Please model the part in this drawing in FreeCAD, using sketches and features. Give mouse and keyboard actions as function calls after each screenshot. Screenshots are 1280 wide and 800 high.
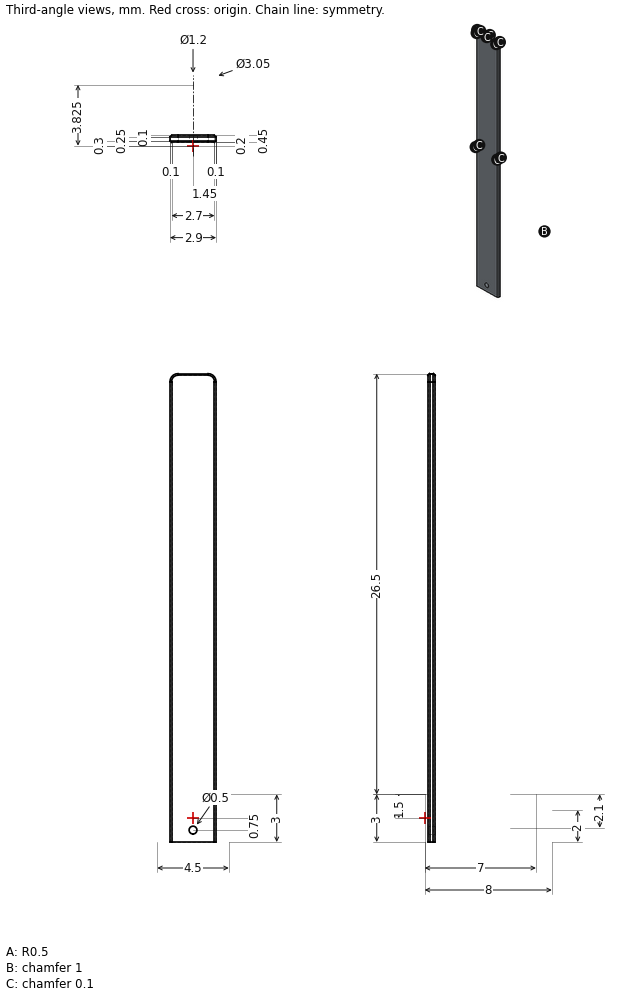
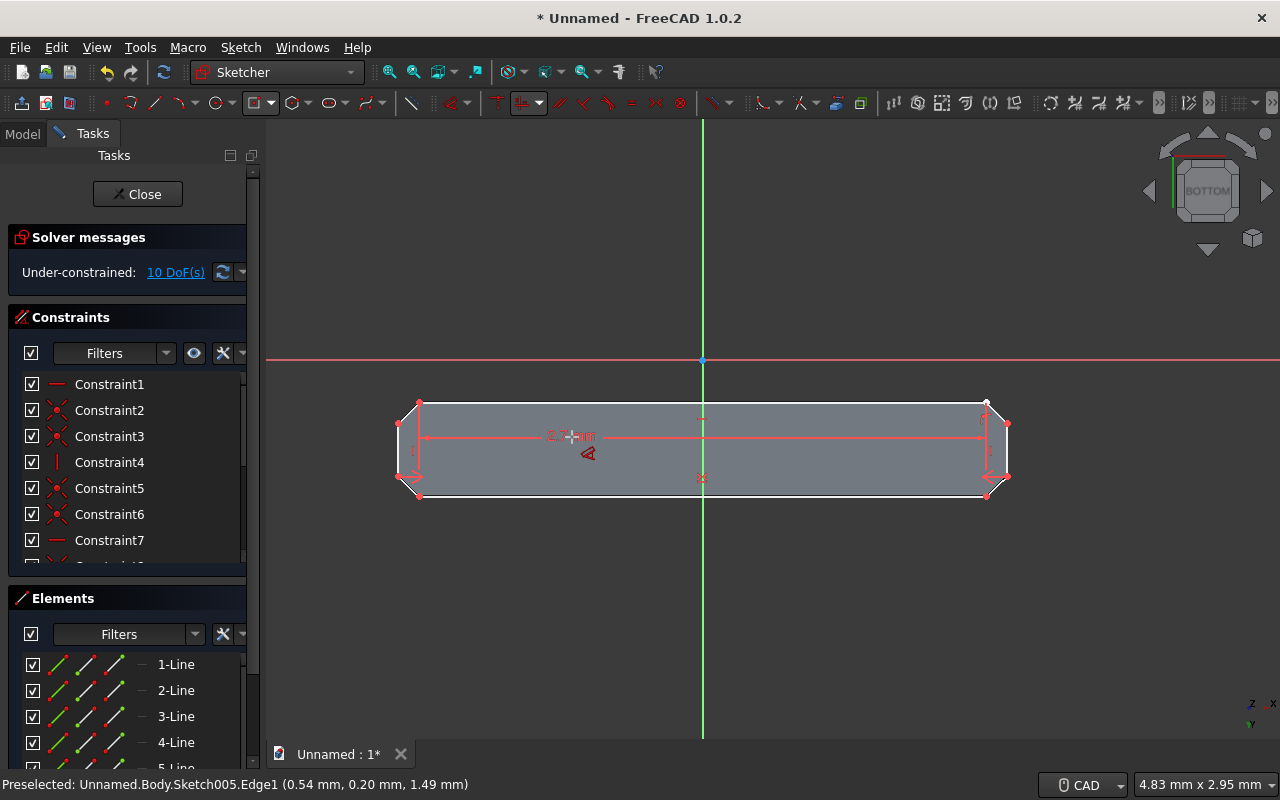
click(589, 497)
click(572, 531)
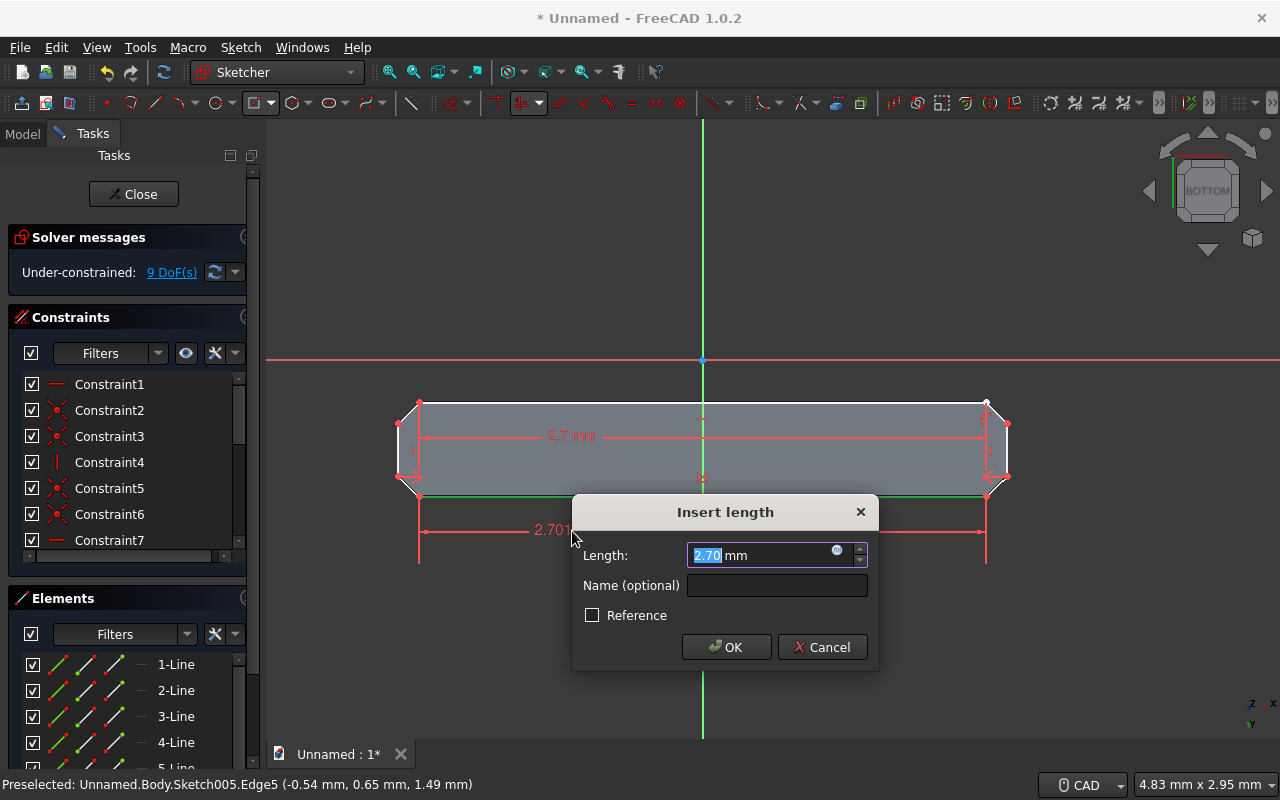
text(2.7)
key(Return)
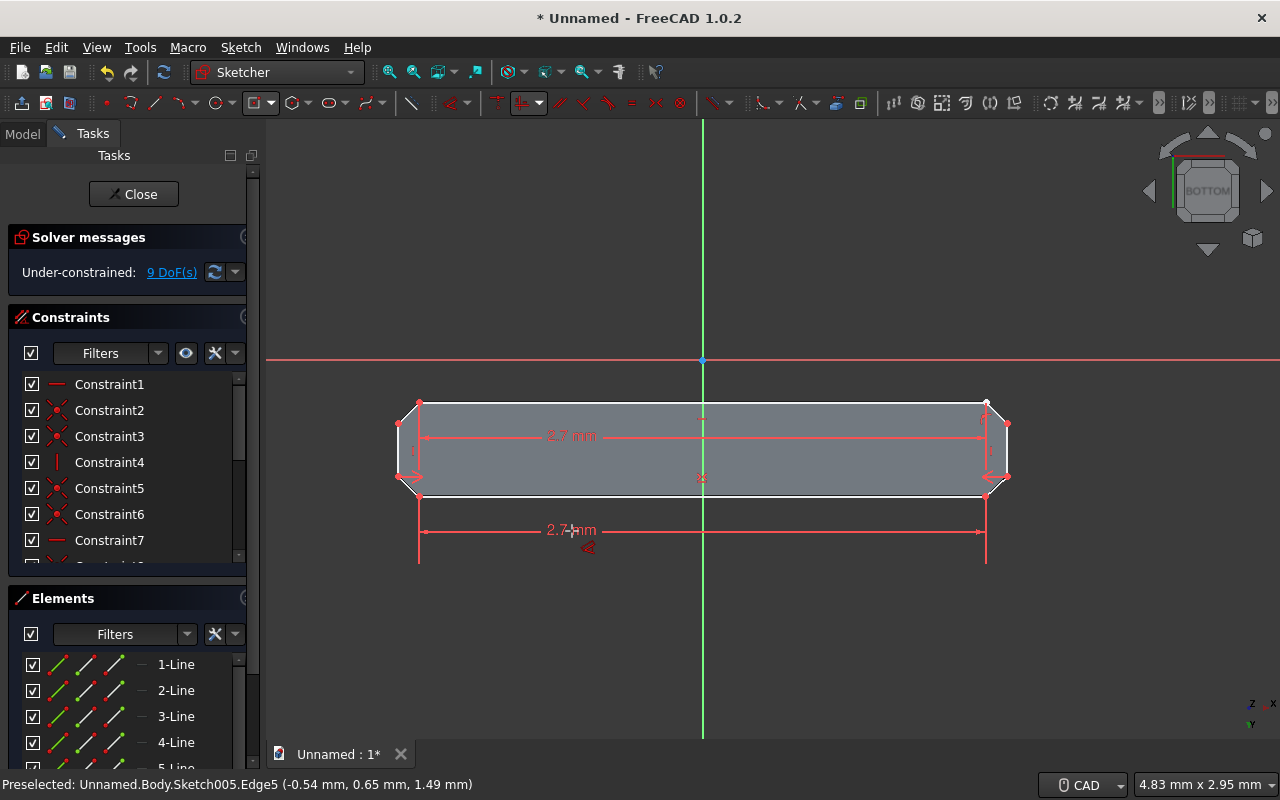
click(398, 440)
click(364, 450)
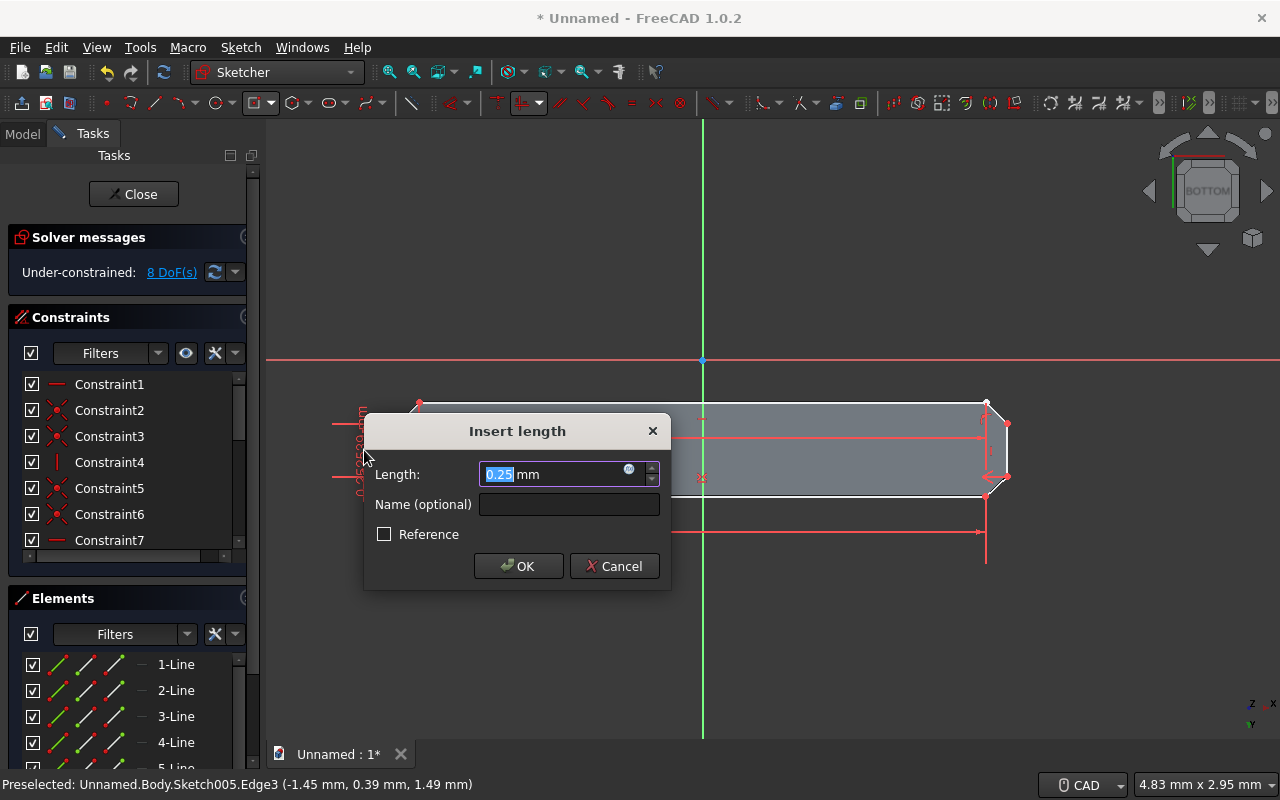
text(0.25)
key(Return)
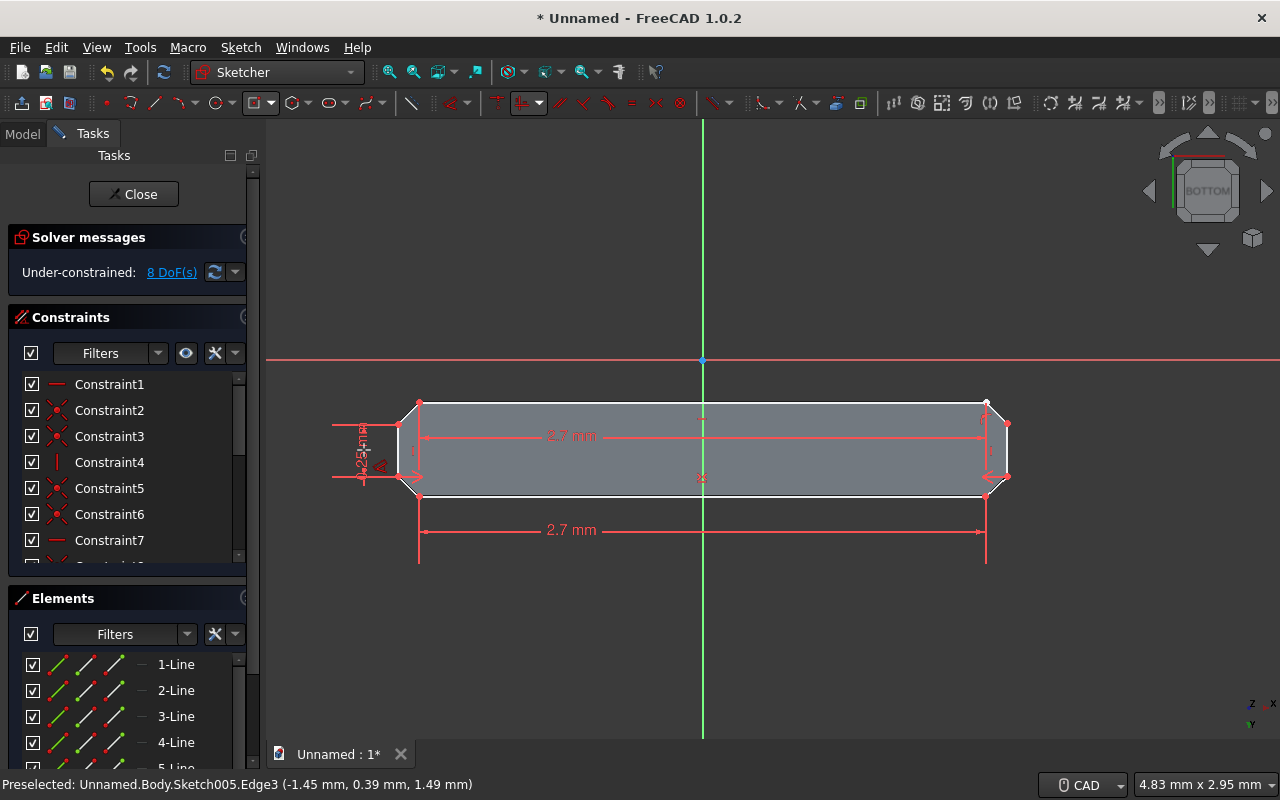
click(1007, 461)
click(1041, 450)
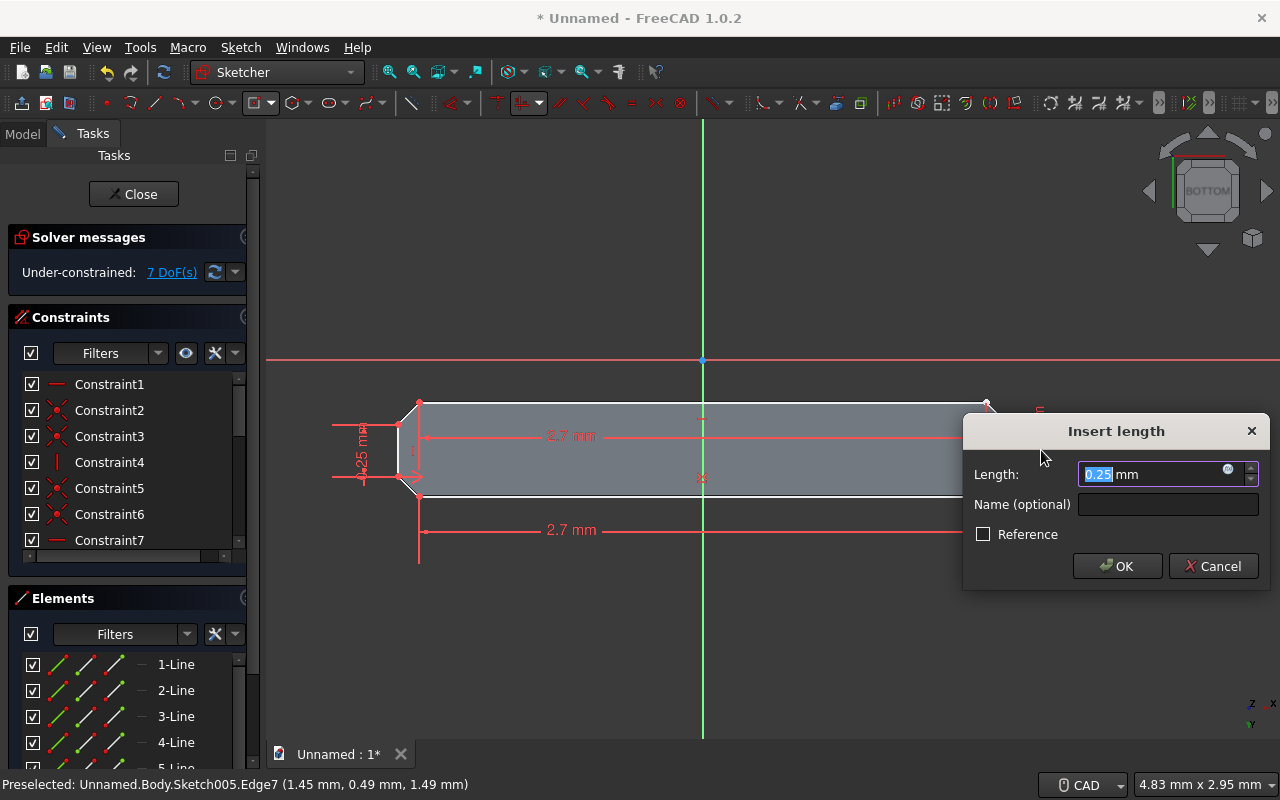
text(0.25)
key(Return)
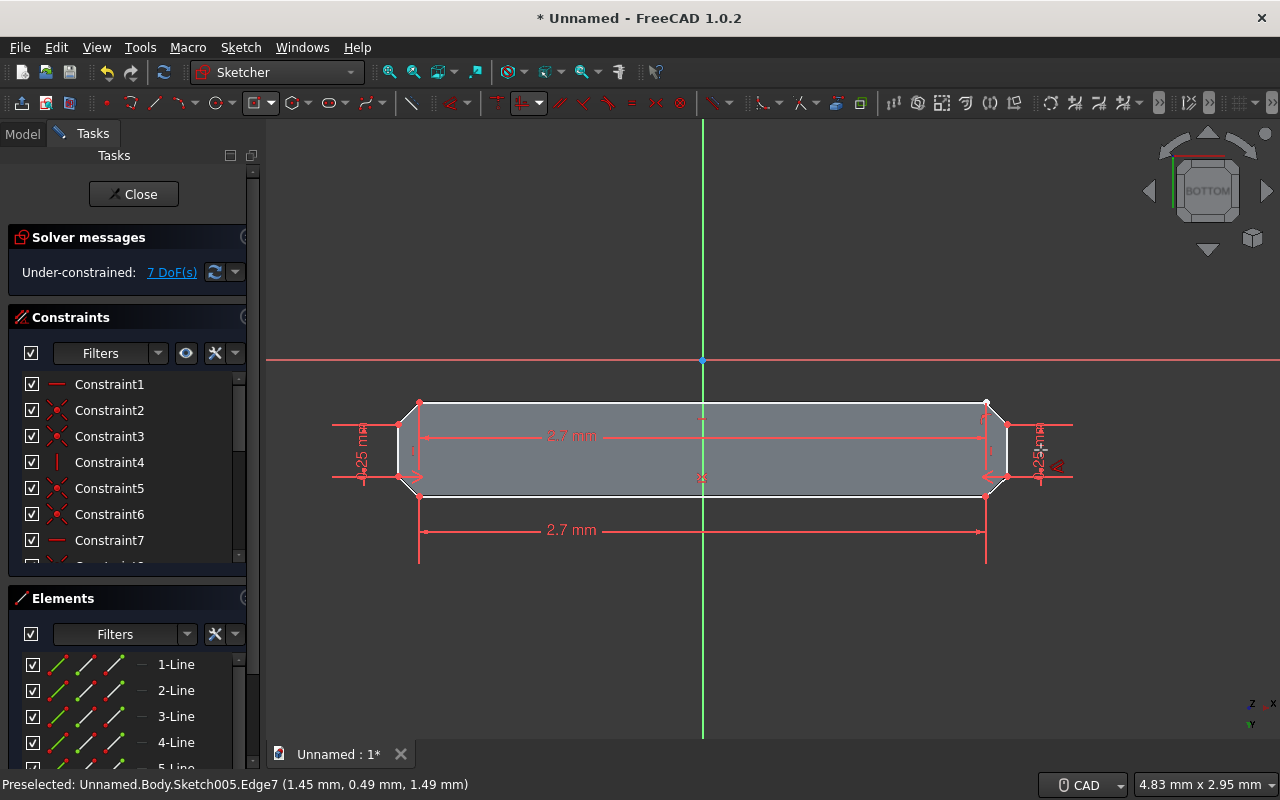
click(986, 403)
click(1020, 382)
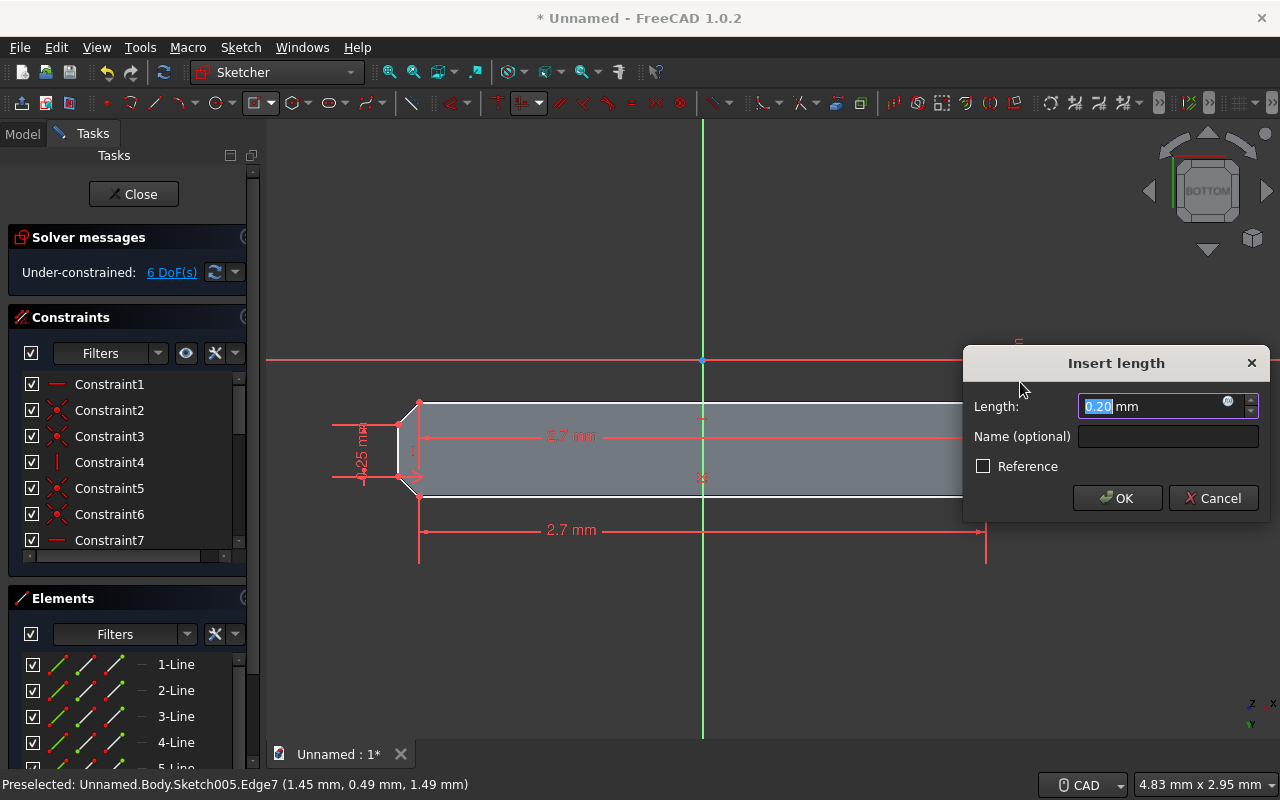
text(0.2)
key(Return)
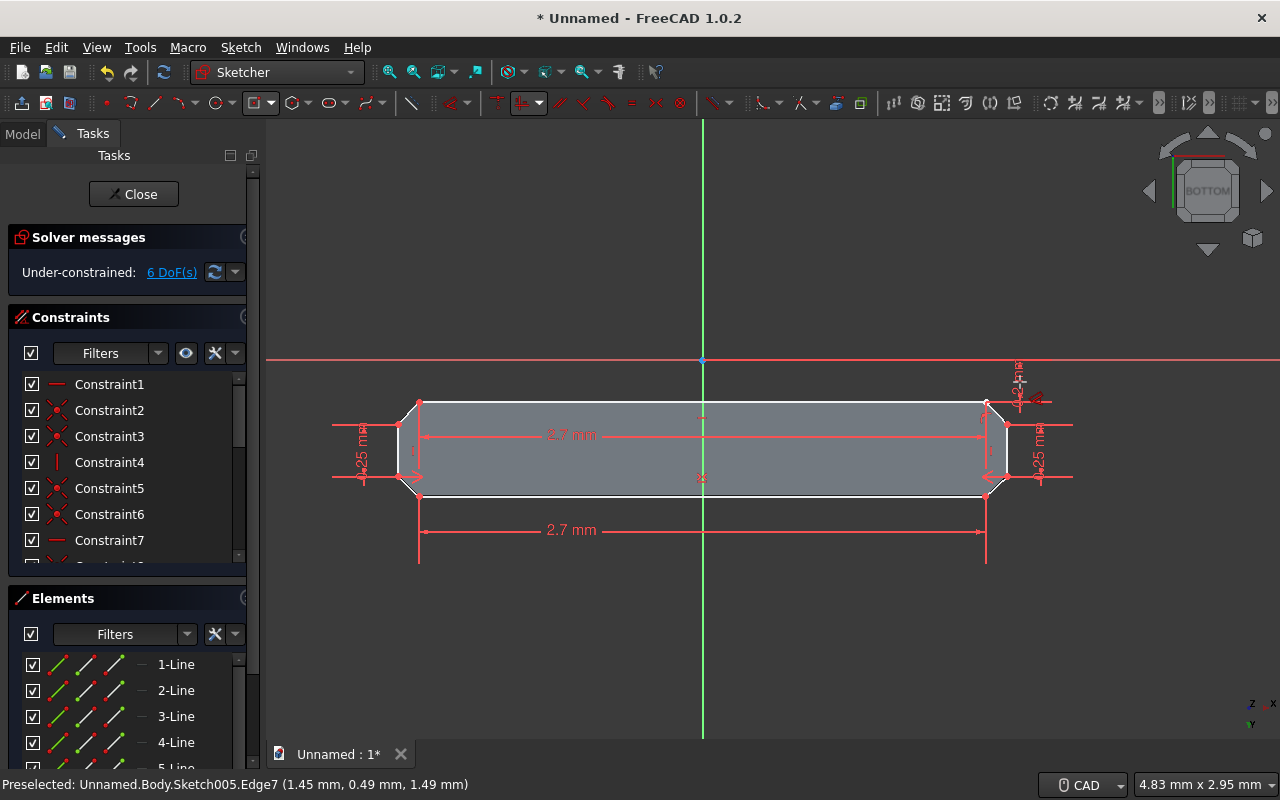
click(398, 425)
click(364, 392)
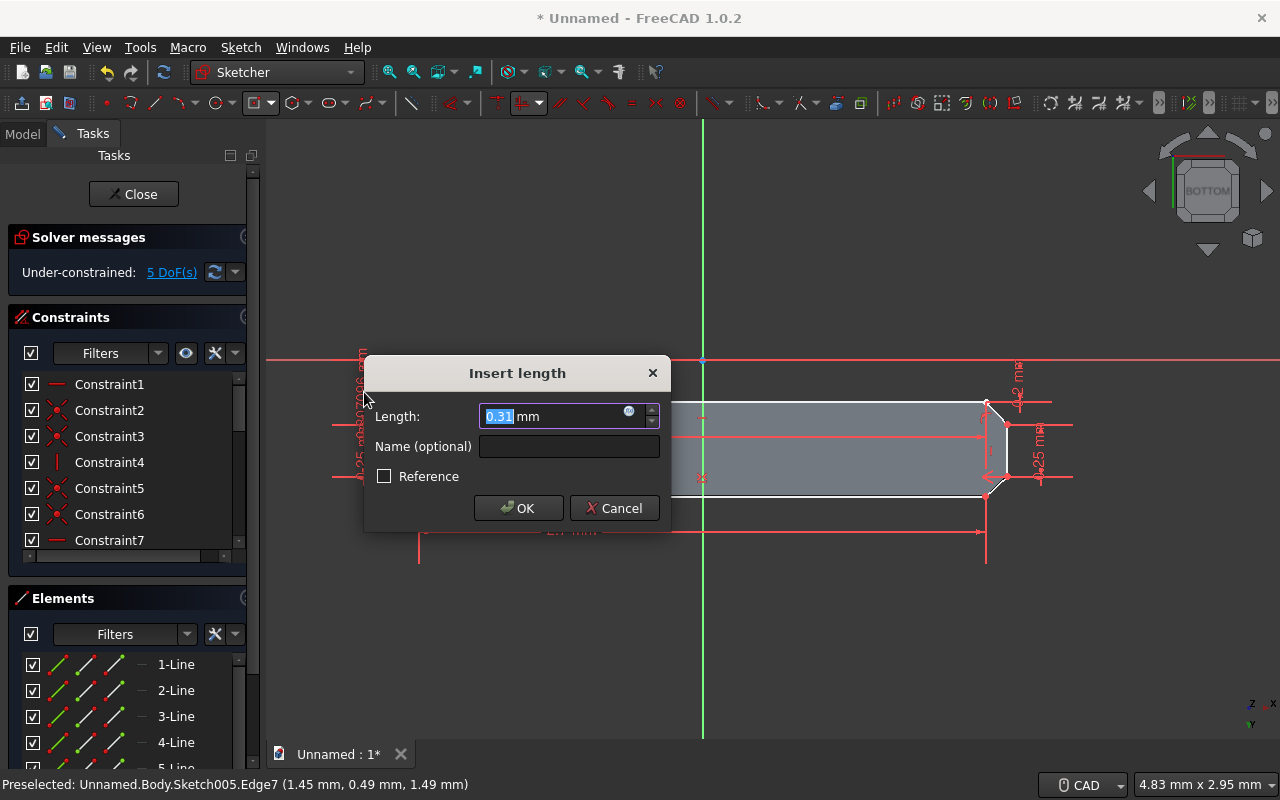
text(0.3)
key(Return)